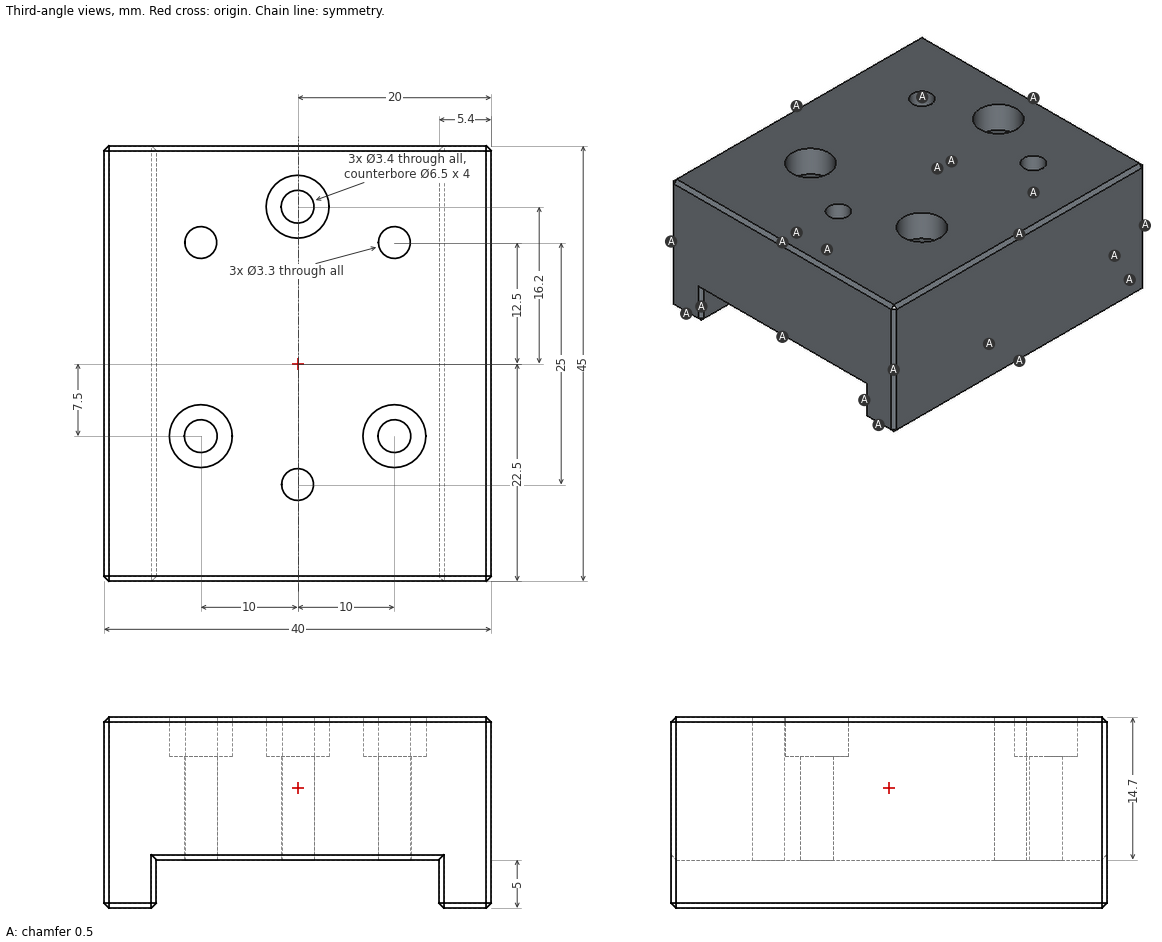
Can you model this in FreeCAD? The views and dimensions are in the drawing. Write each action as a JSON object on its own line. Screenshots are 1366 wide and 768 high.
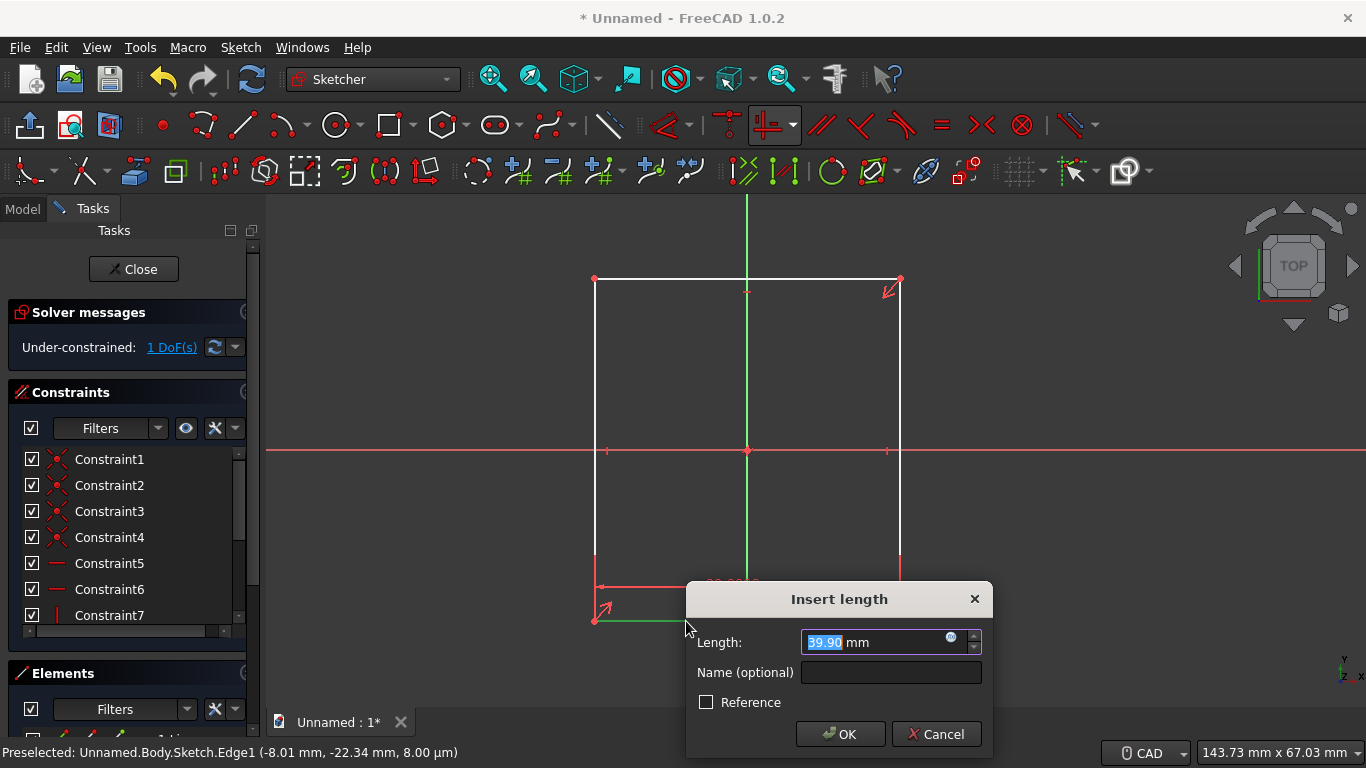
{"action": "type", "text": "40"}
{"action": "key", "text": "Return"}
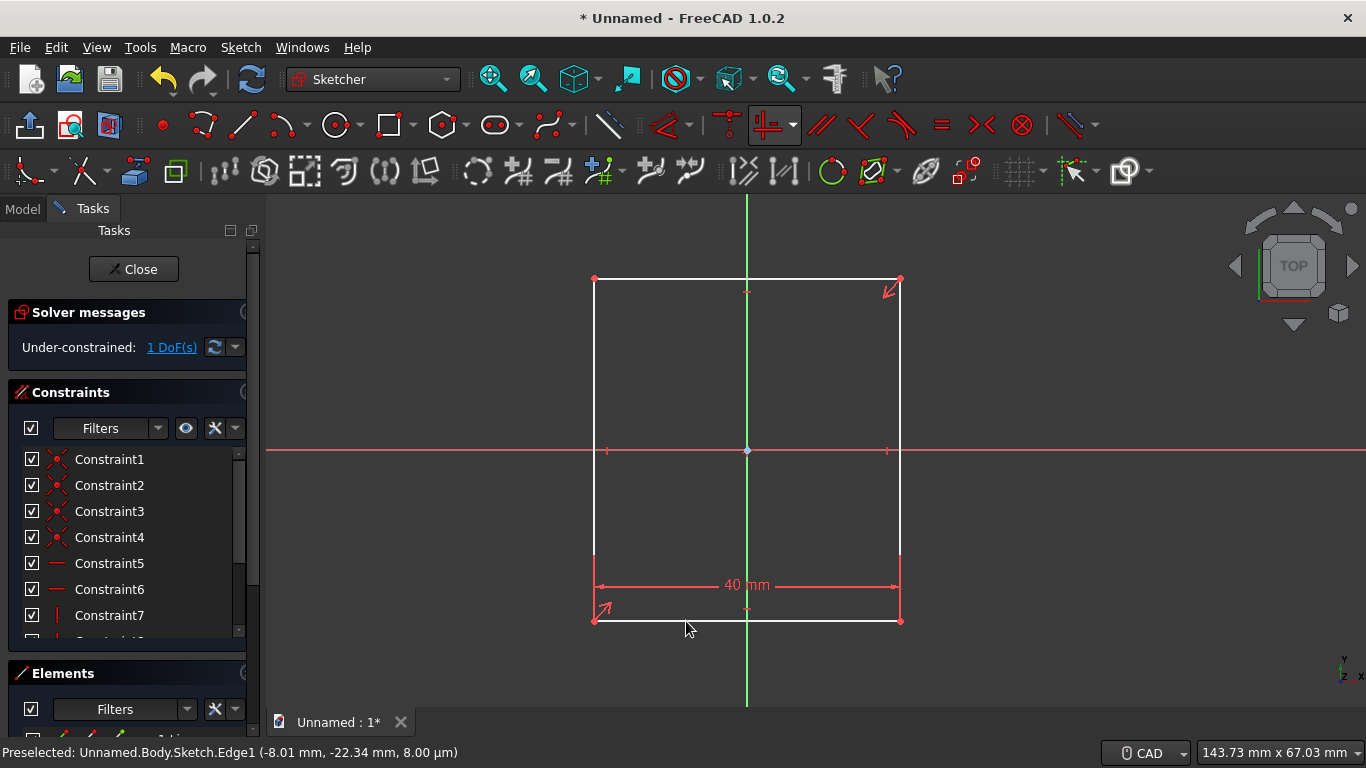
{"action": "left_click", "coordinate": [900, 518]}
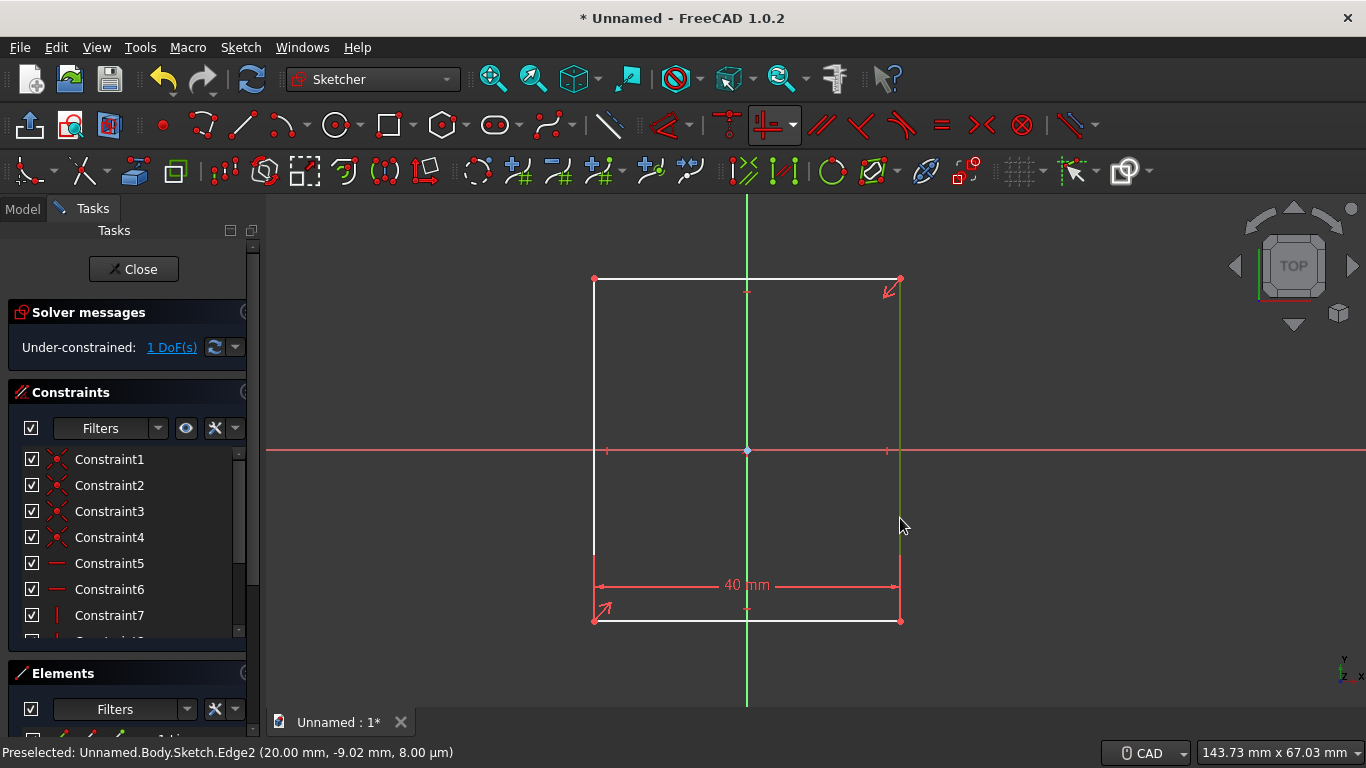
{"action": "left_click", "coordinate": [692, 126]}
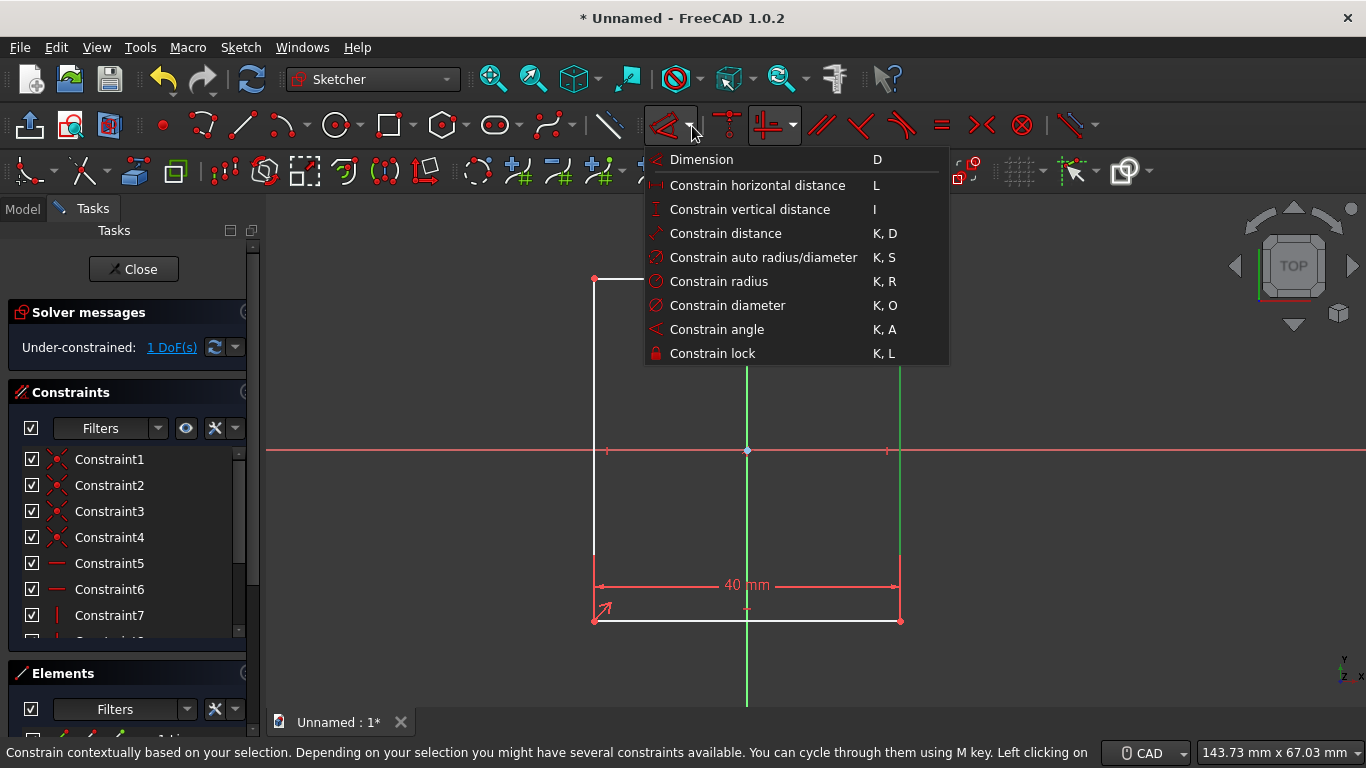
{"action": "left_click", "coordinate": [797, 209]}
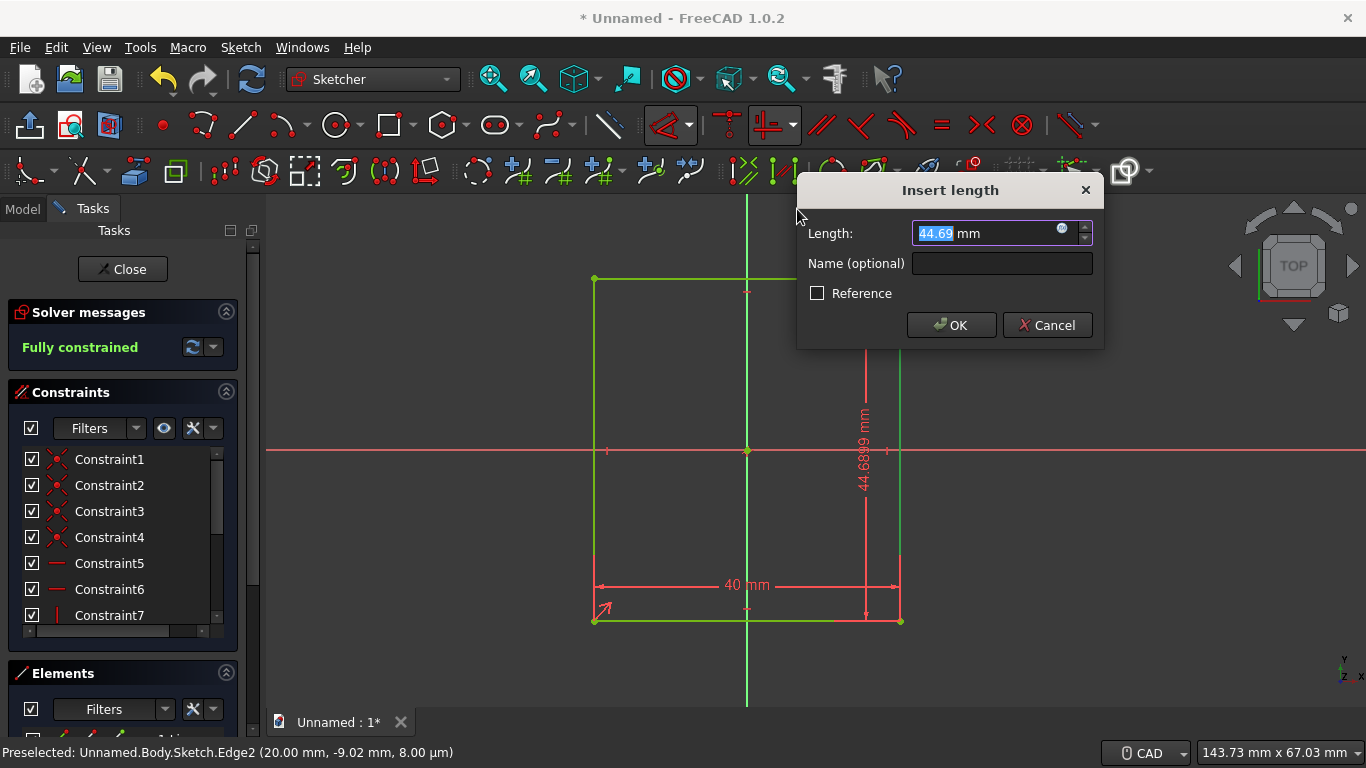
{"action": "type", "text": "45"}
{"action": "key", "text": "Return"}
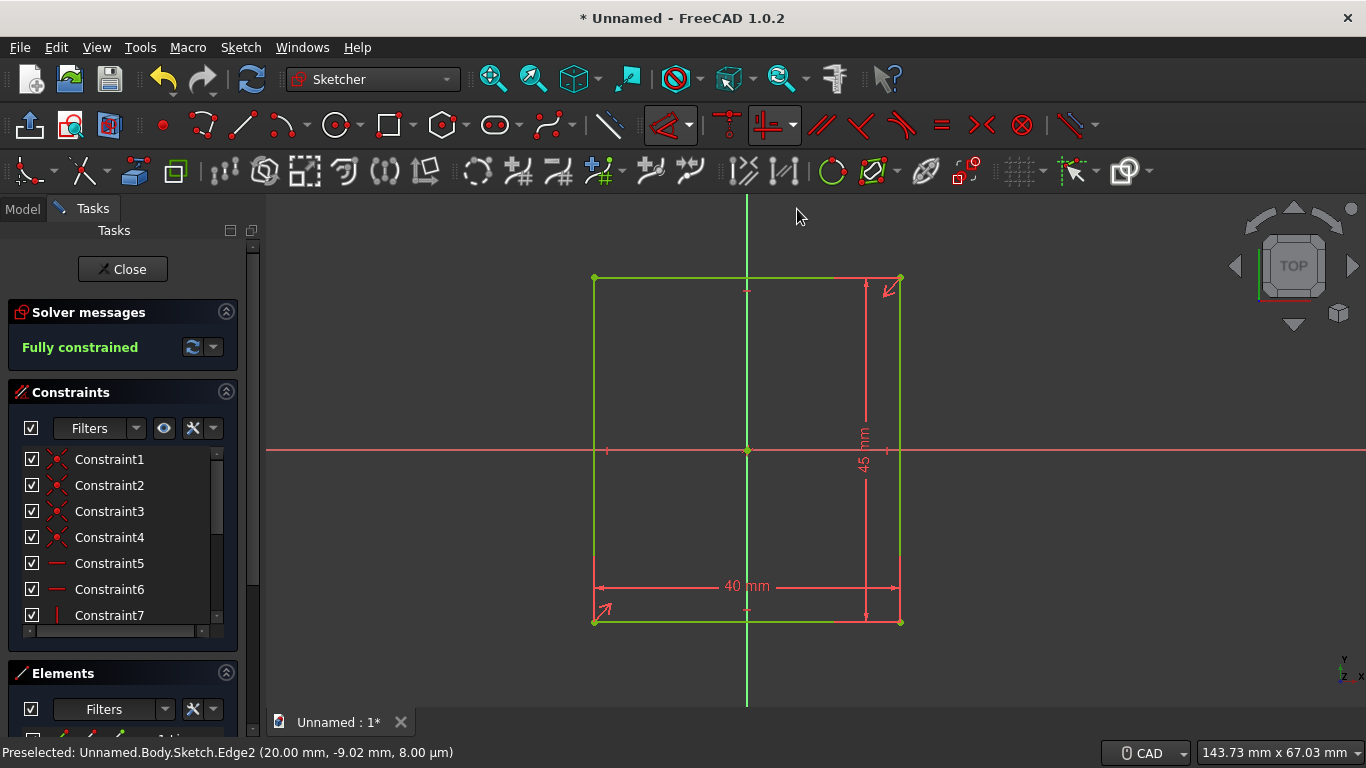
{"action": "left_click", "coordinate": [123, 269]}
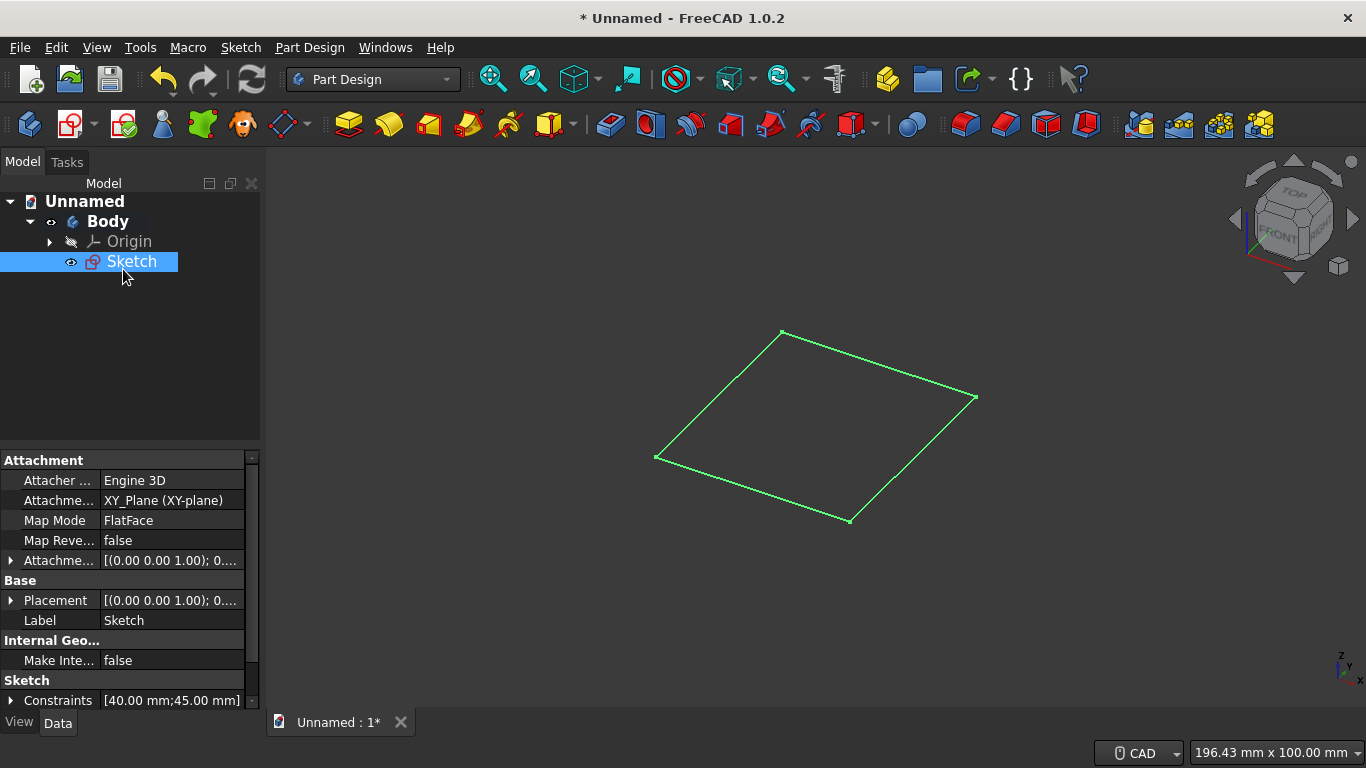
{"action": "left_click", "coordinate": [350, 124]}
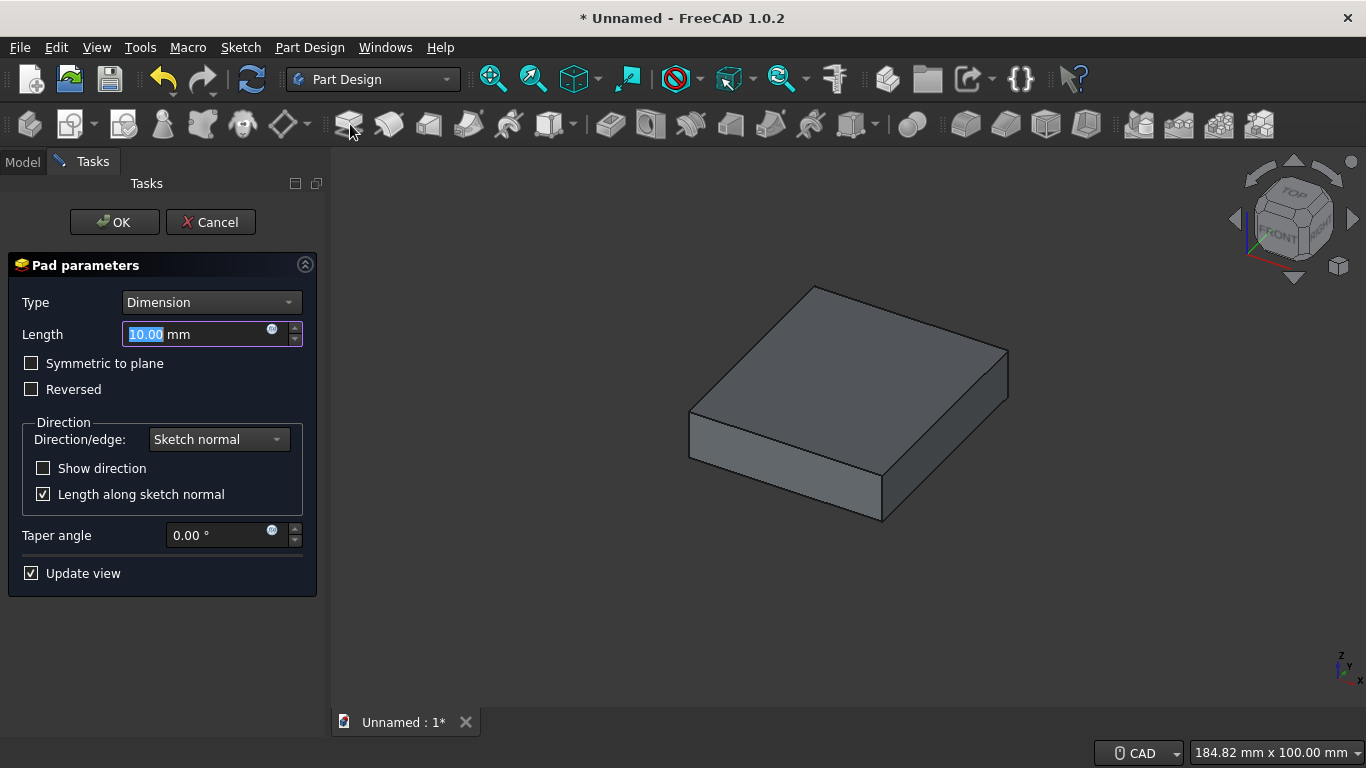
{"action": "type", "text": "14.7"}
{"action": "key", "text": "Tab"}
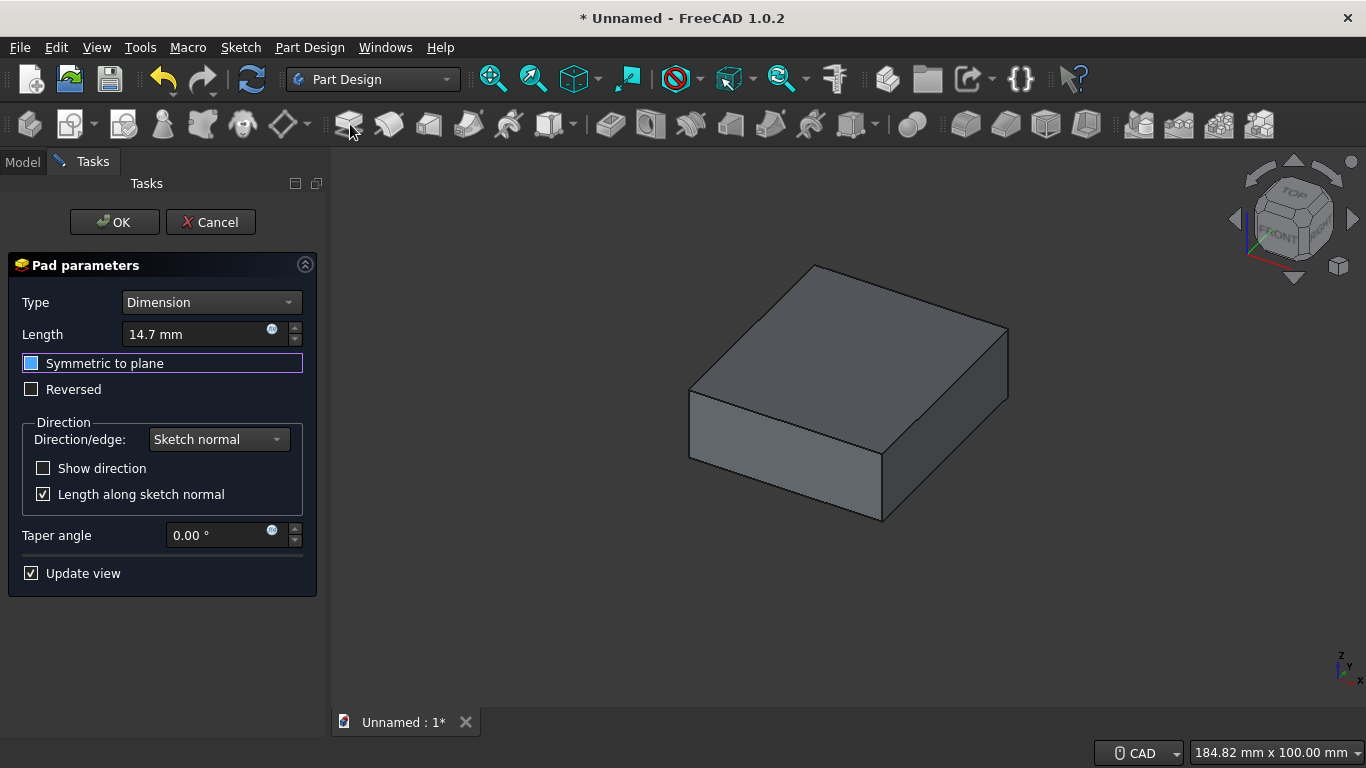
{"action": "left_click", "coordinate": [30, 363]}